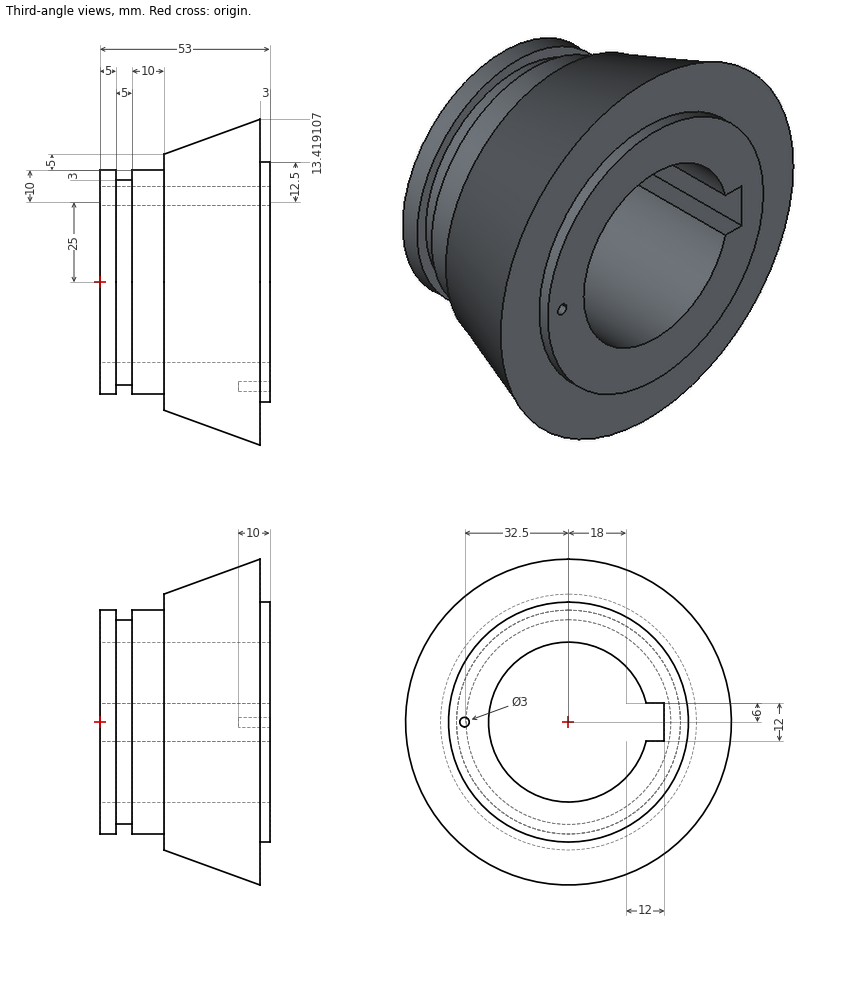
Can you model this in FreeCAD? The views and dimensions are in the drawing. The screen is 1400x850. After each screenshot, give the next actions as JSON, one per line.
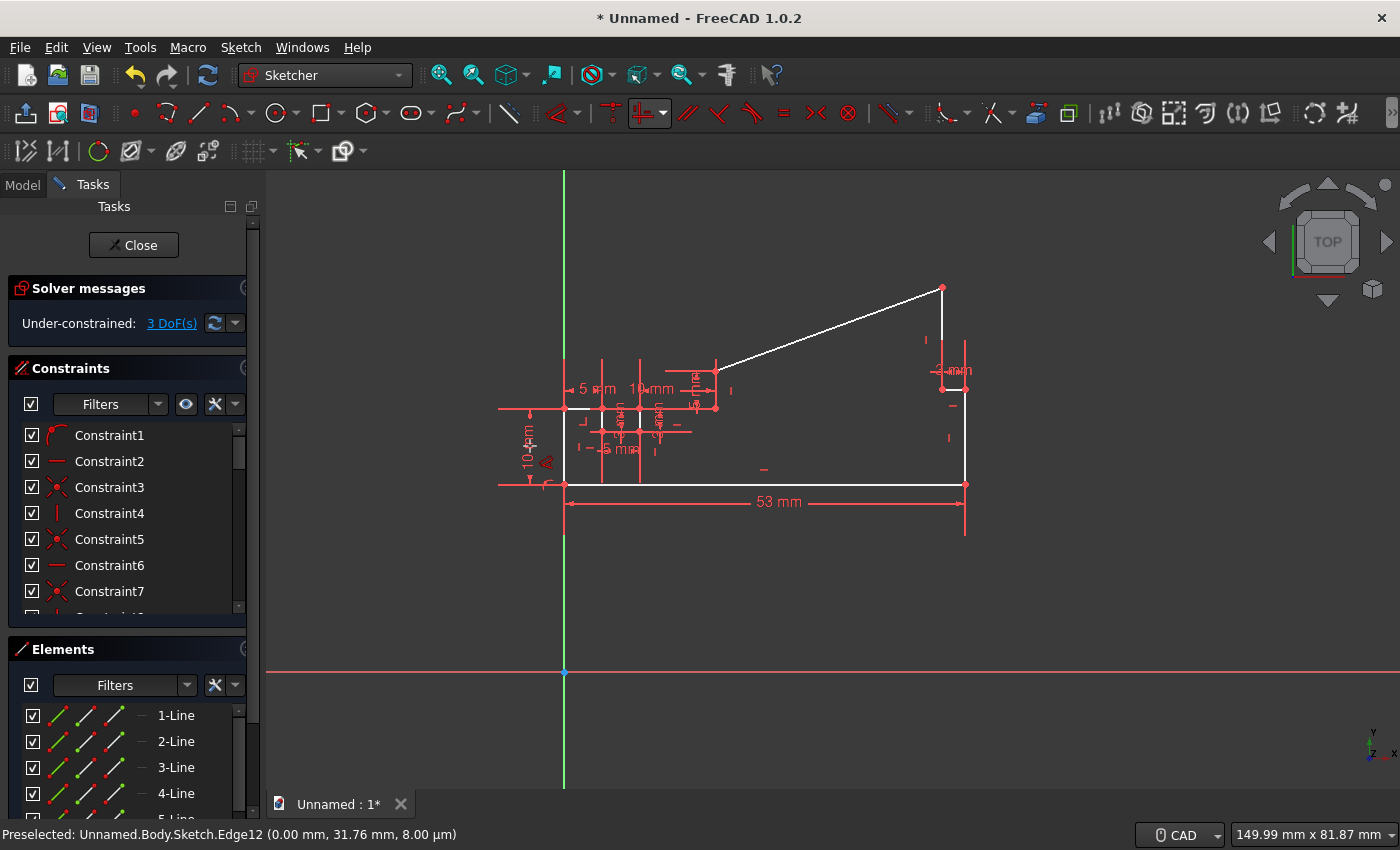
{"action": "left_click", "coordinate": [564, 485]}
{"action": "left_click", "coordinate": [530, 578]}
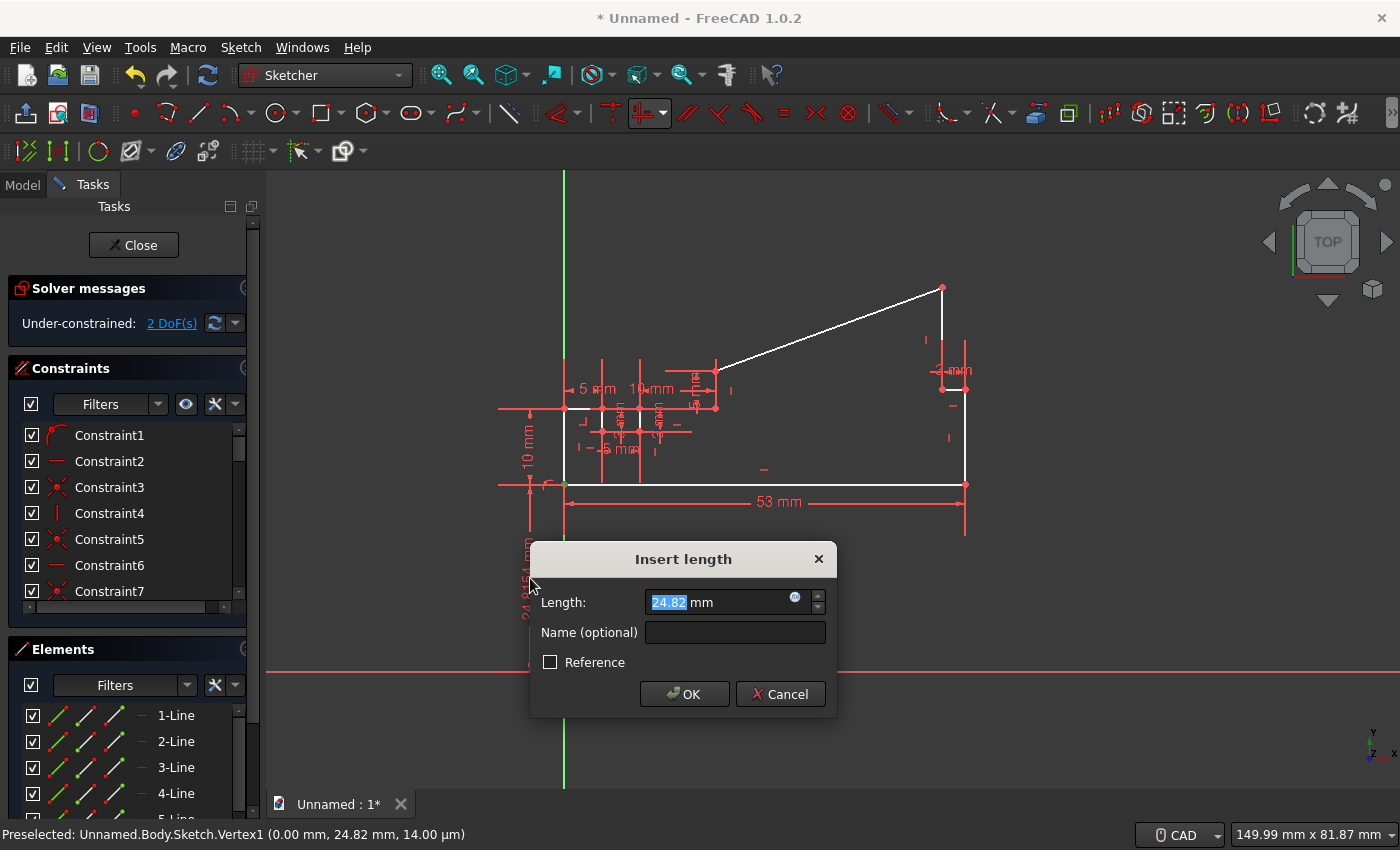
{"action": "type", "text": "25"}
{"action": "key", "text": "Return"}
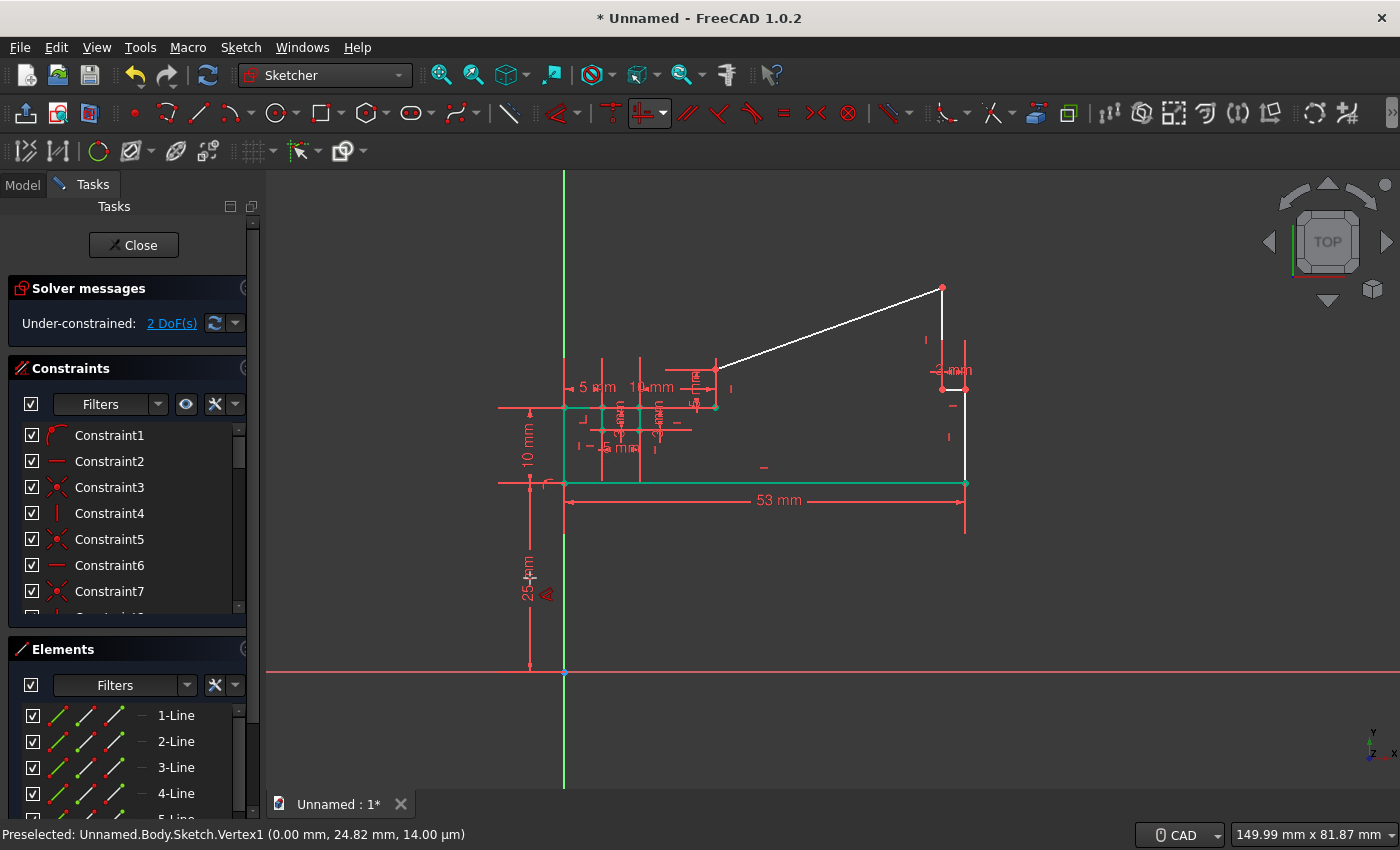
{"action": "left_click", "coordinate": [965, 455]}
{"action": "left_click", "coordinate": [999, 437]}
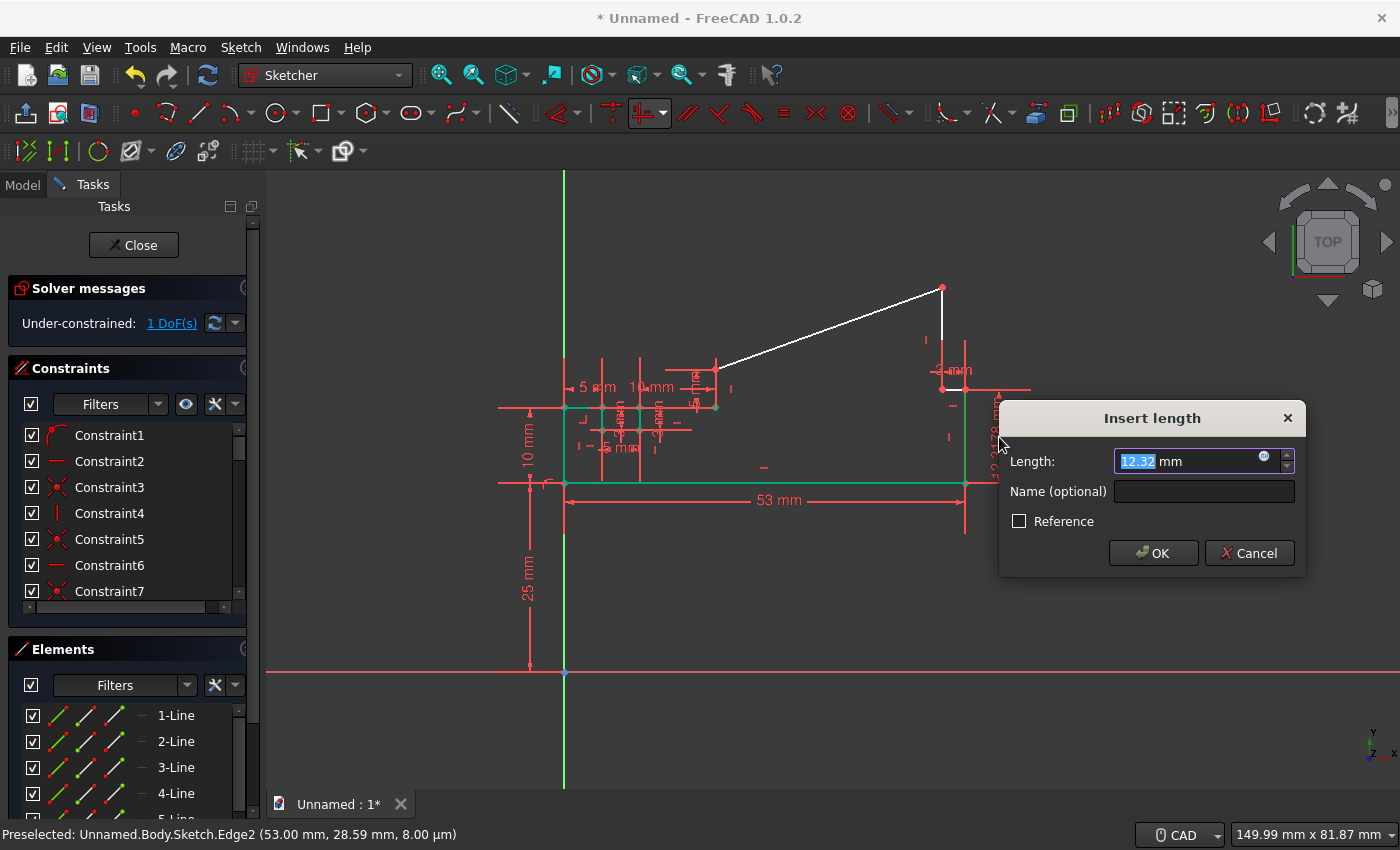
{"action": "type", "text": "12.5"}
{"action": "key", "text": "Return"}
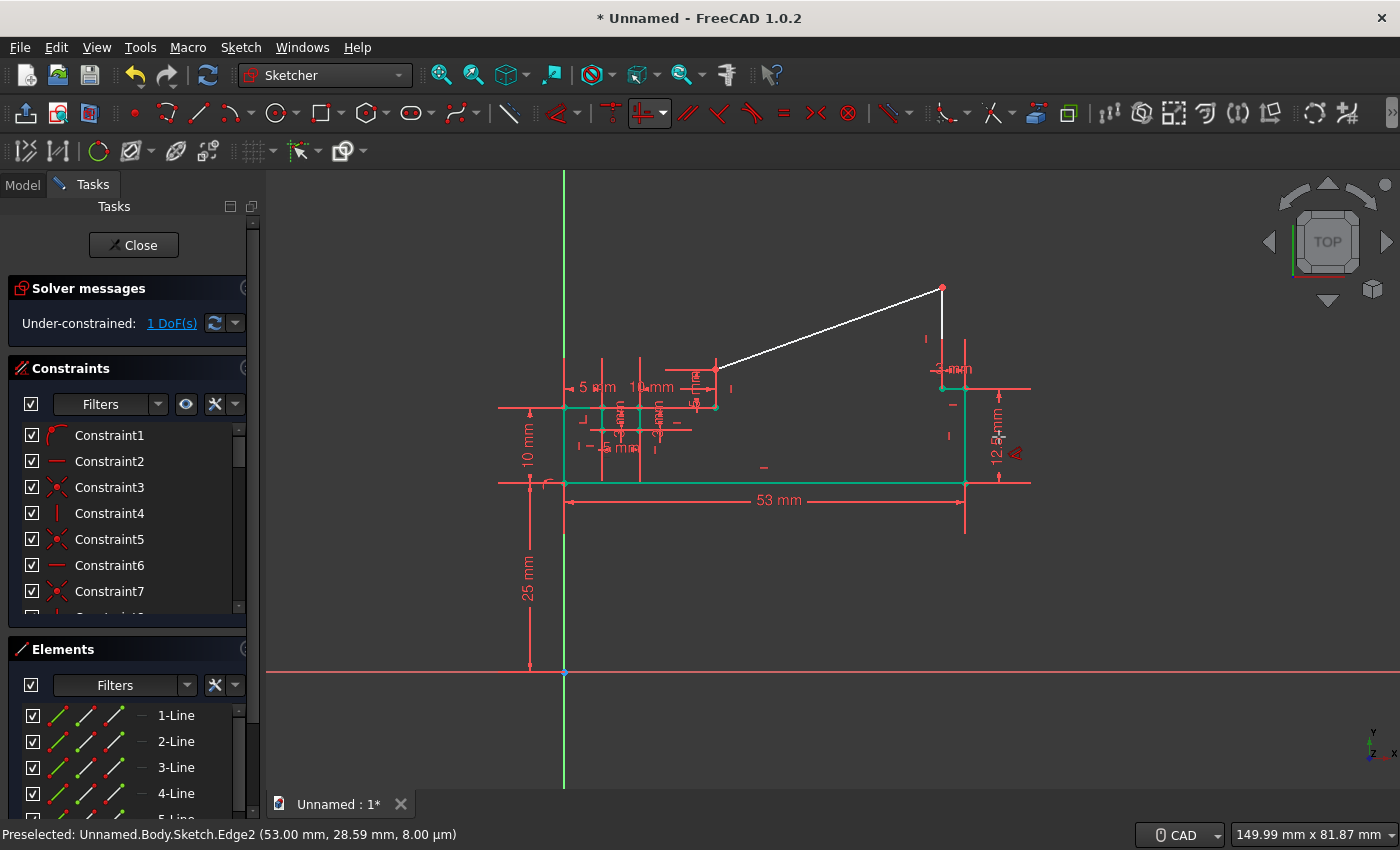
{"action": "left_click", "coordinate": [942, 358]}
{"action": "left_click", "coordinate": [976, 338]}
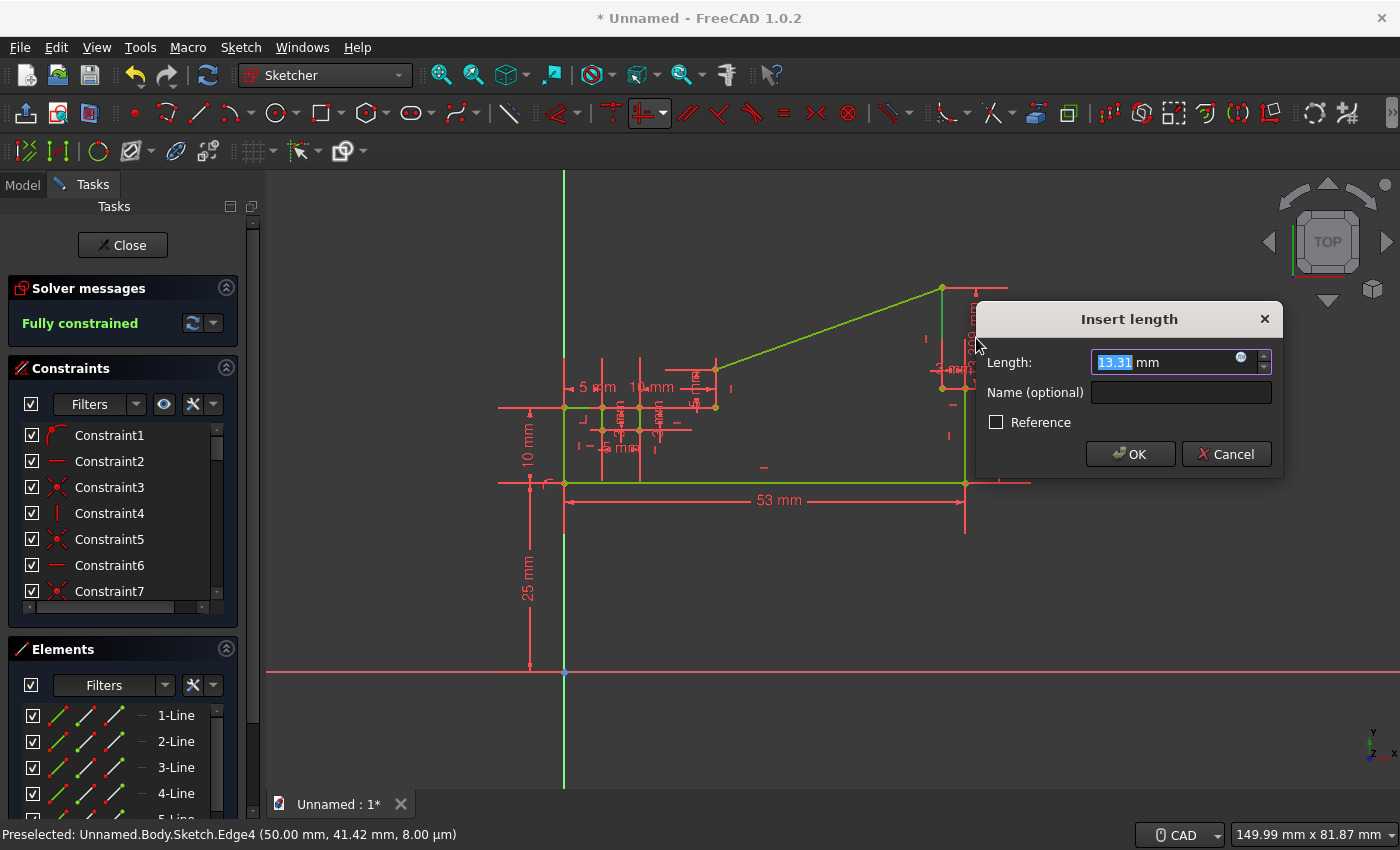
{"action": "type", "text": "13.419107"}
{"action": "key", "text": "Return"}
{"action": "key", "text": "Escape"}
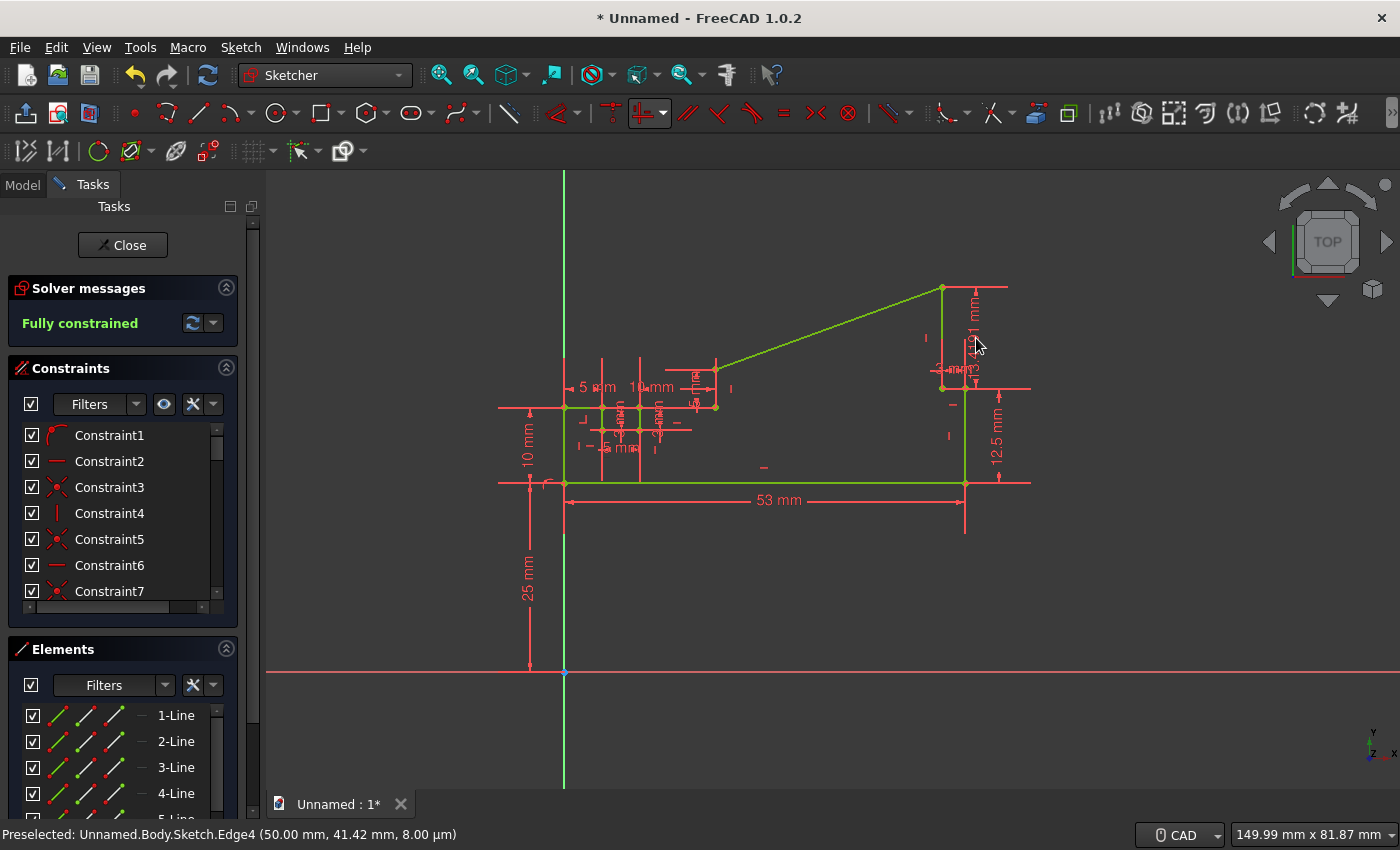
{"action": "left_click", "coordinate": [123, 245]}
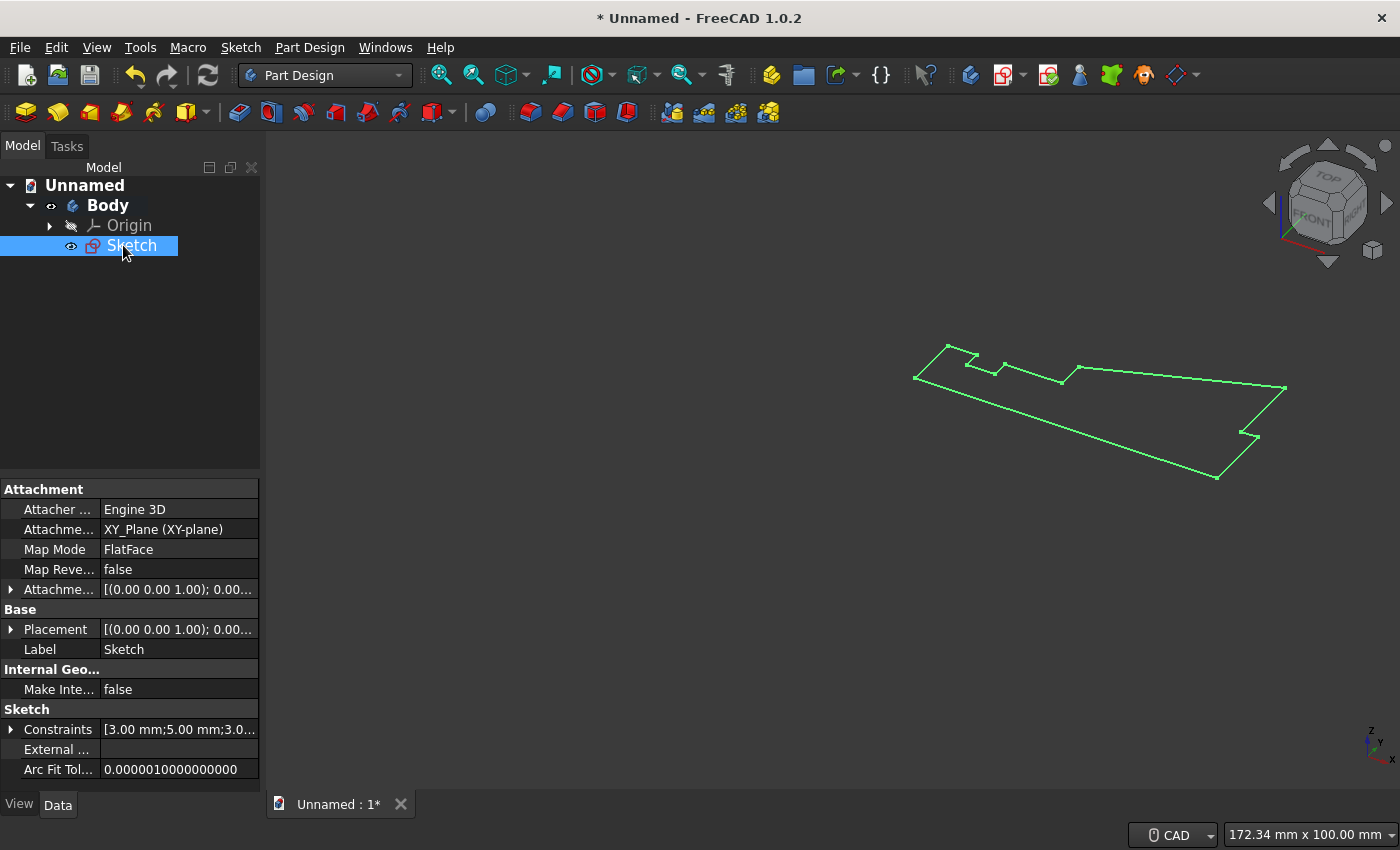
{"action": "left_click", "coordinate": [58, 112]}